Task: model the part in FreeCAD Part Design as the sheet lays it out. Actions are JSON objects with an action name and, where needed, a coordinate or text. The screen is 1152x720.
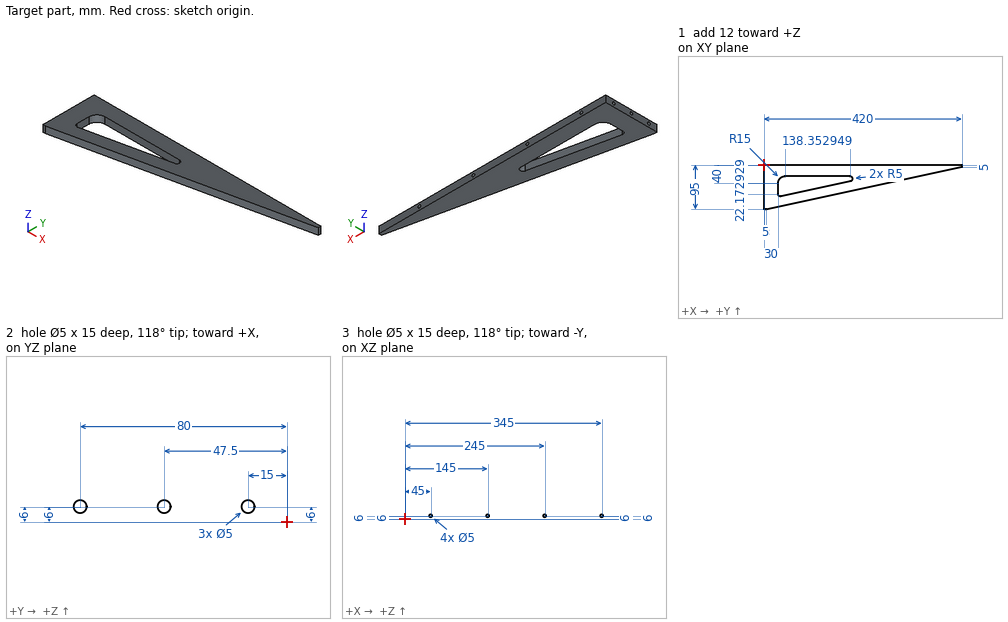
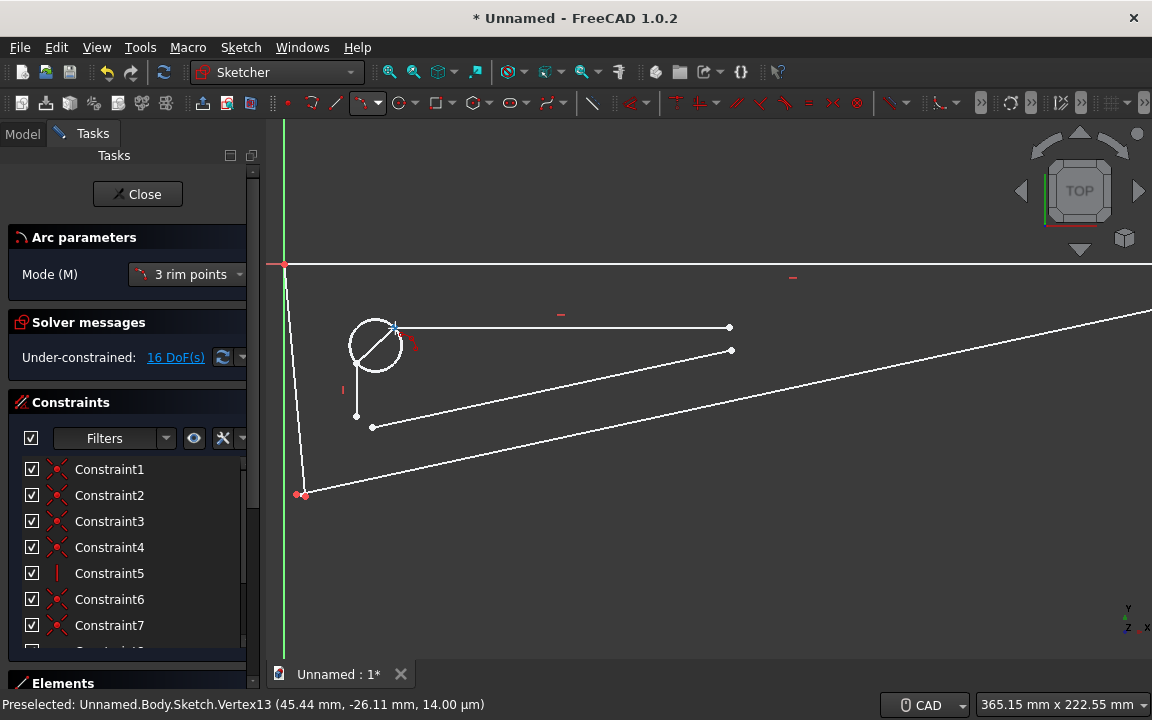
{"action": "scroll", "coordinate": [368, 336], "scroll_direction": "up", "scroll_amount": 2}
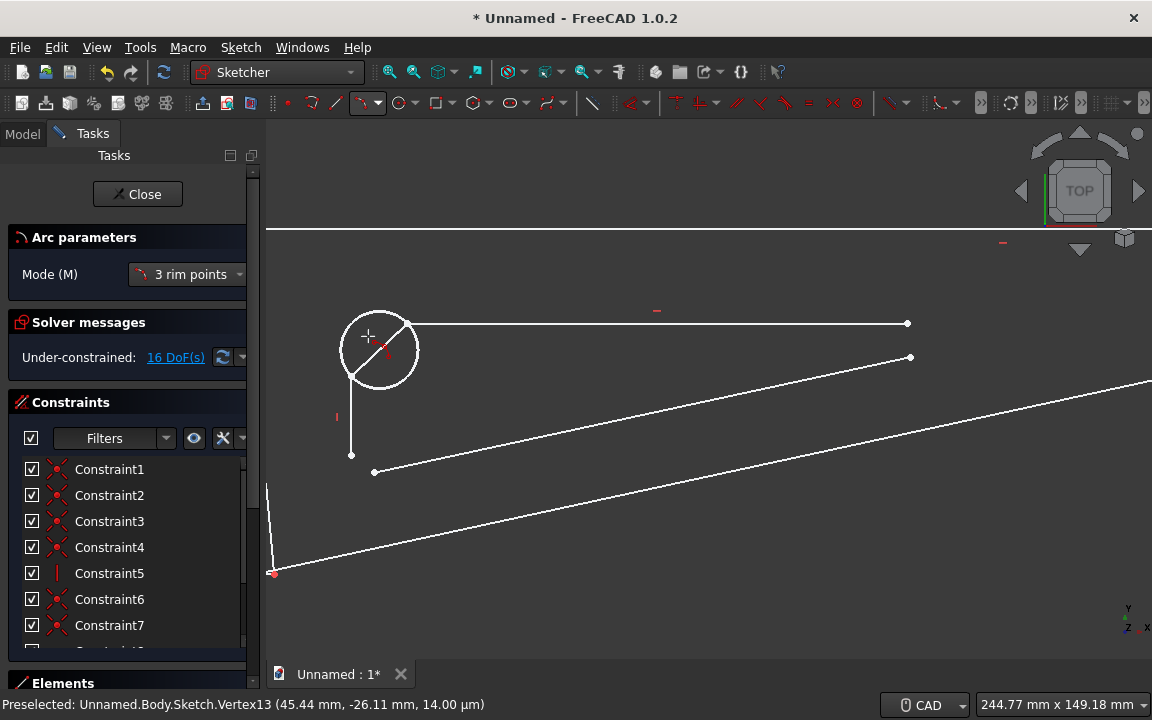
{"action": "left_click", "coordinate": [368, 335]}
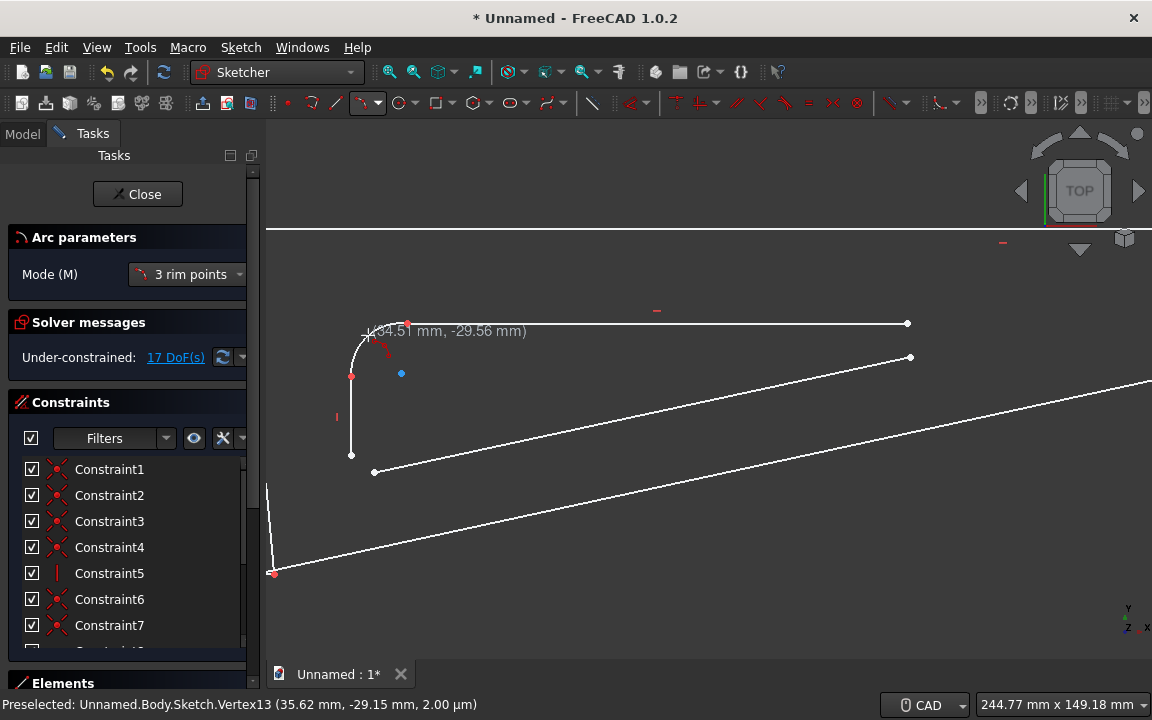
{"action": "left_click", "coordinate": [907, 324]}
{"action": "left_click", "coordinate": [911, 357]}
{"action": "left_click", "coordinate": [925, 336]}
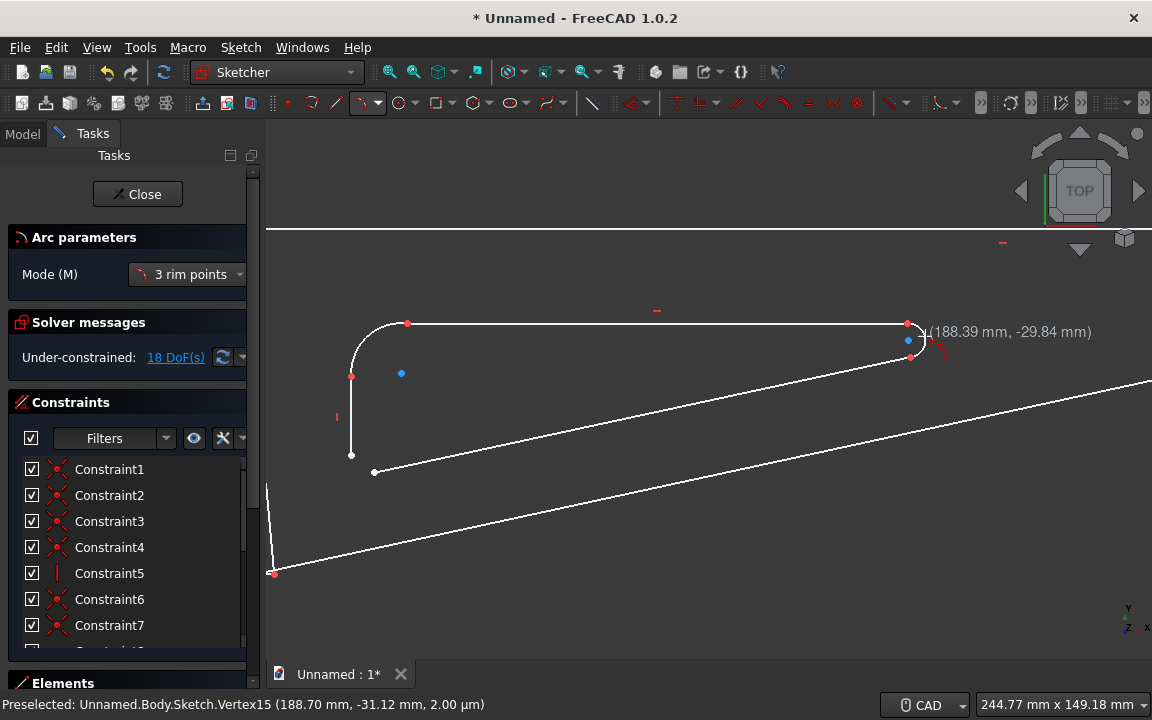
{"action": "left_click", "coordinate": [374, 473]}
{"action": "left_click", "coordinate": [351, 456]}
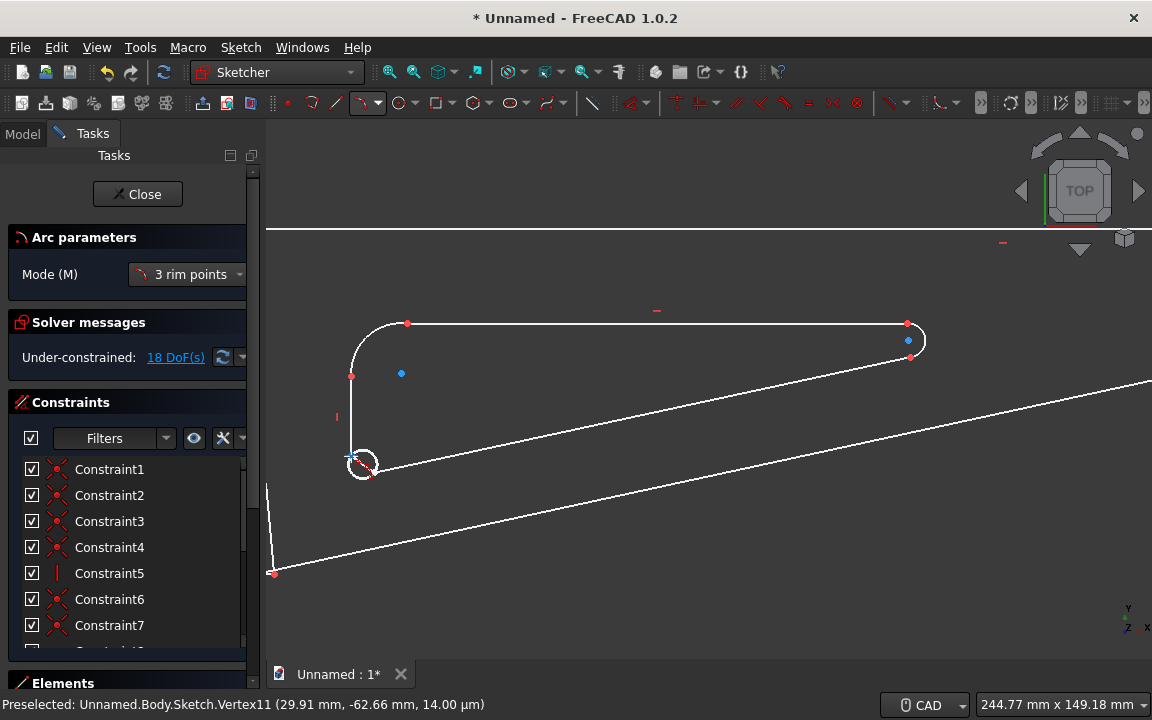
{"action": "scroll", "coordinate": [358, 468], "scroll_direction": "up", "scroll_amount": 5}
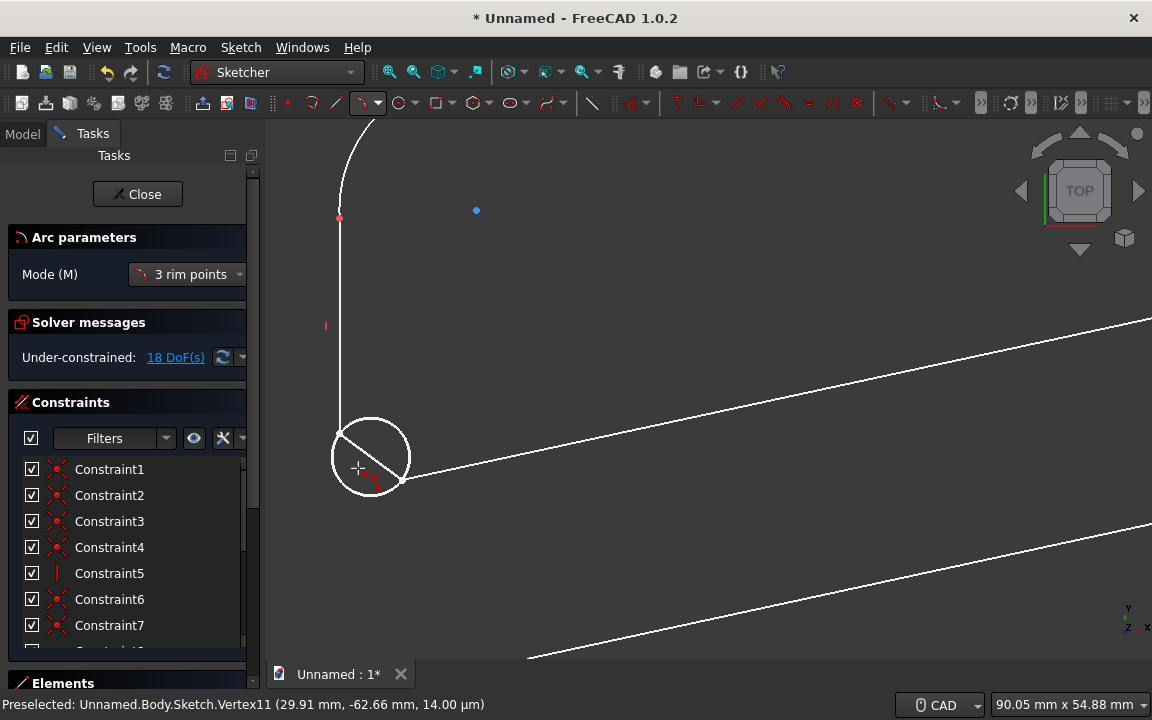
{"action": "left_click", "coordinate": [359, 467]}
{"action": "key", "text": "Escape"}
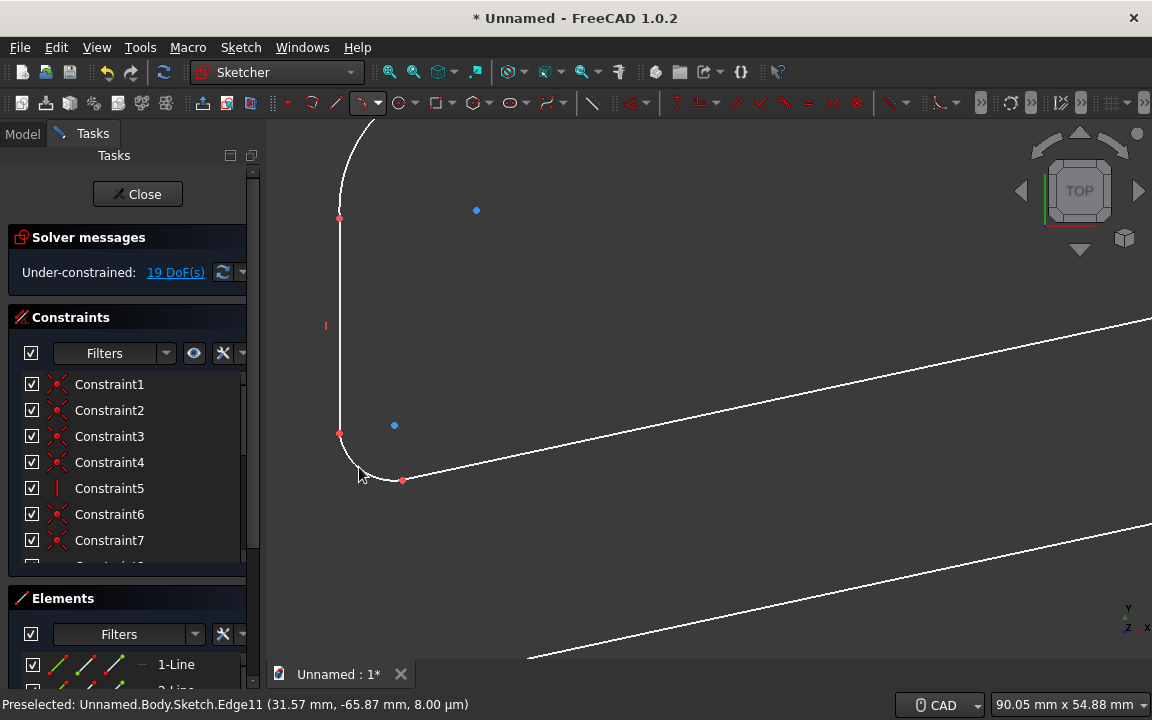
{"action": "scroll", "coordinate": [457, 402], "scroll_direction": "down", "scroll_amount": 11}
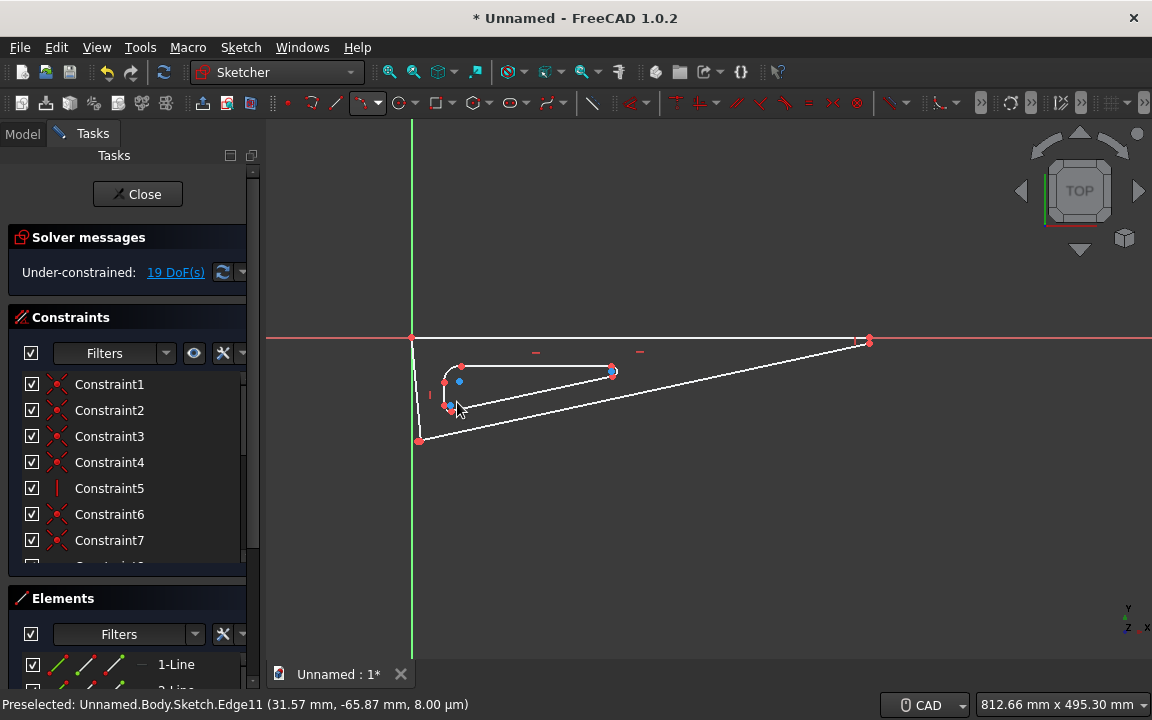
{"action": "scroll", "coordinate": [444, 399], "scroll_direction": "up", "scroll_amount": 4}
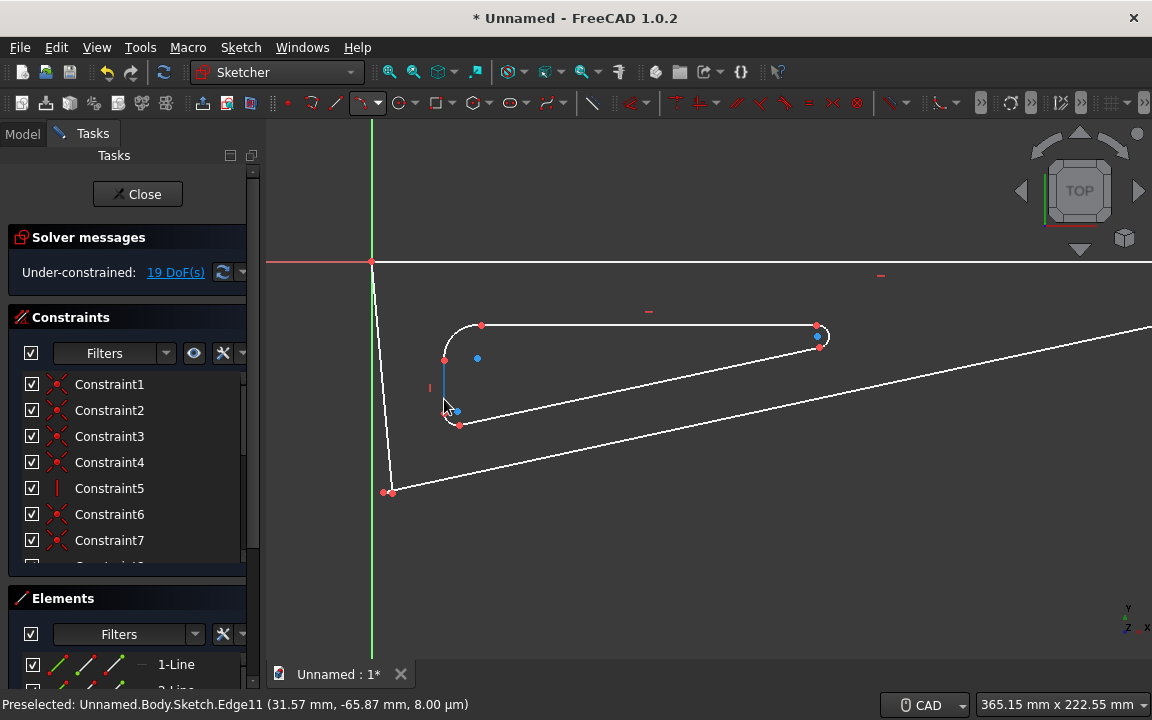
{"action": "left_click", "coordinate": [444, 398]}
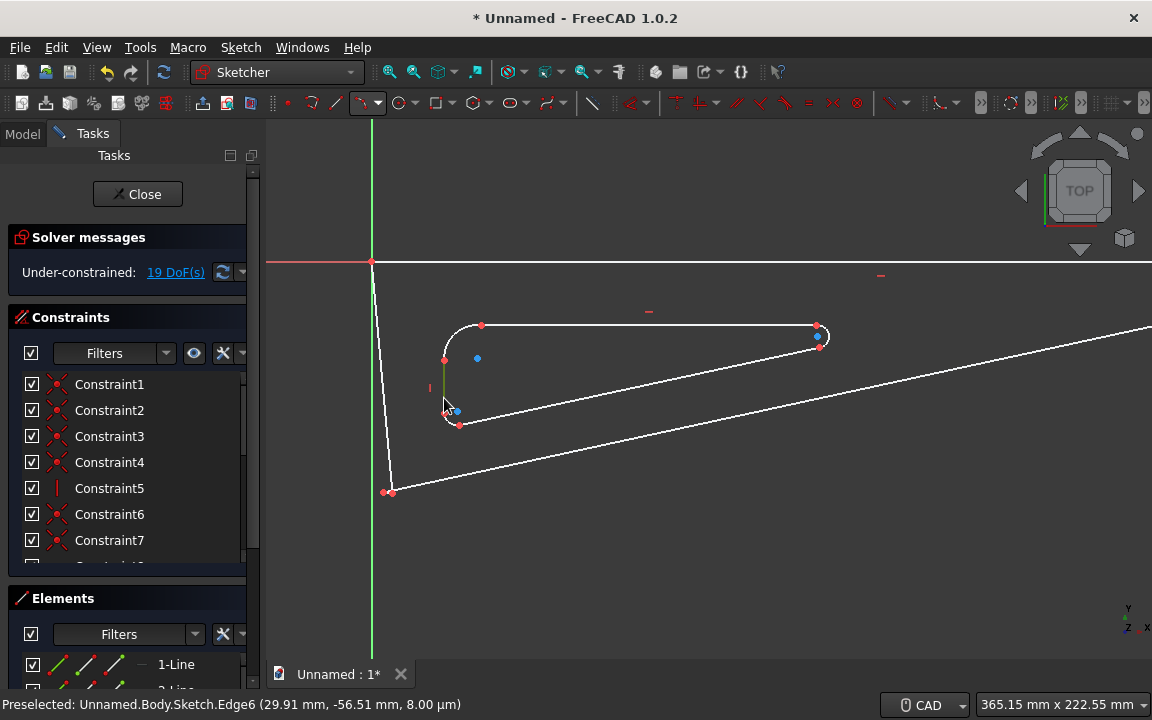
{"action": "left_click", "coordinate": [465, 328]}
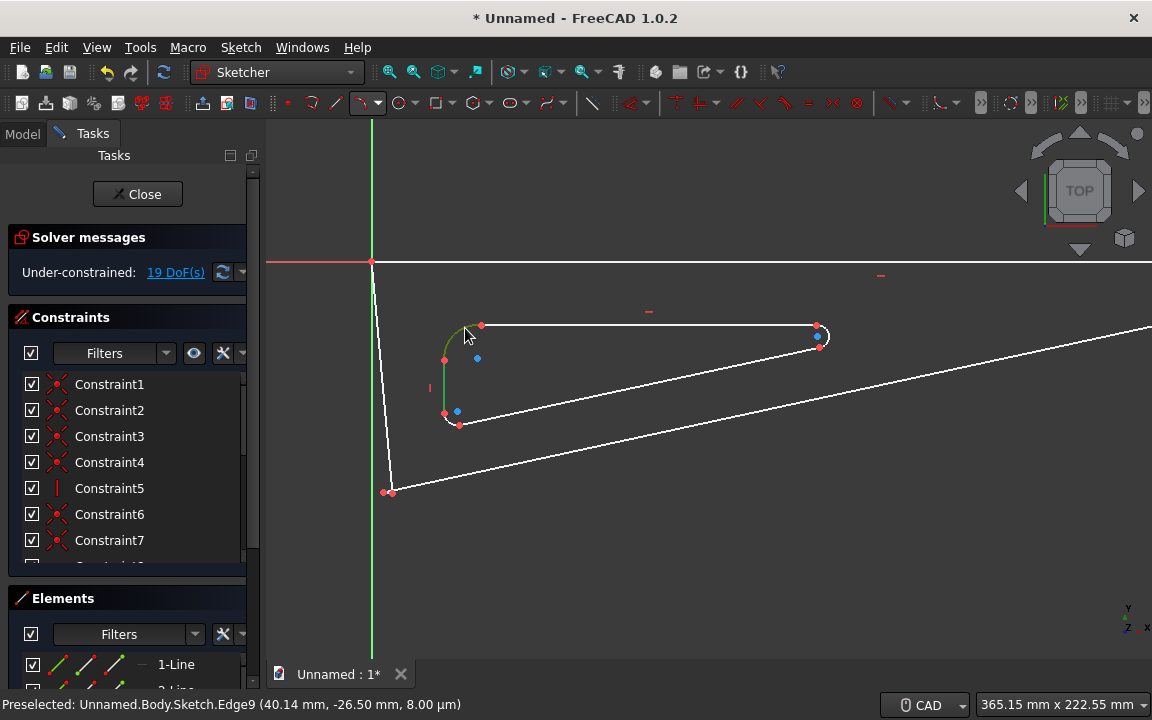
{"action": "left_click", "coordinate": [786, 104]}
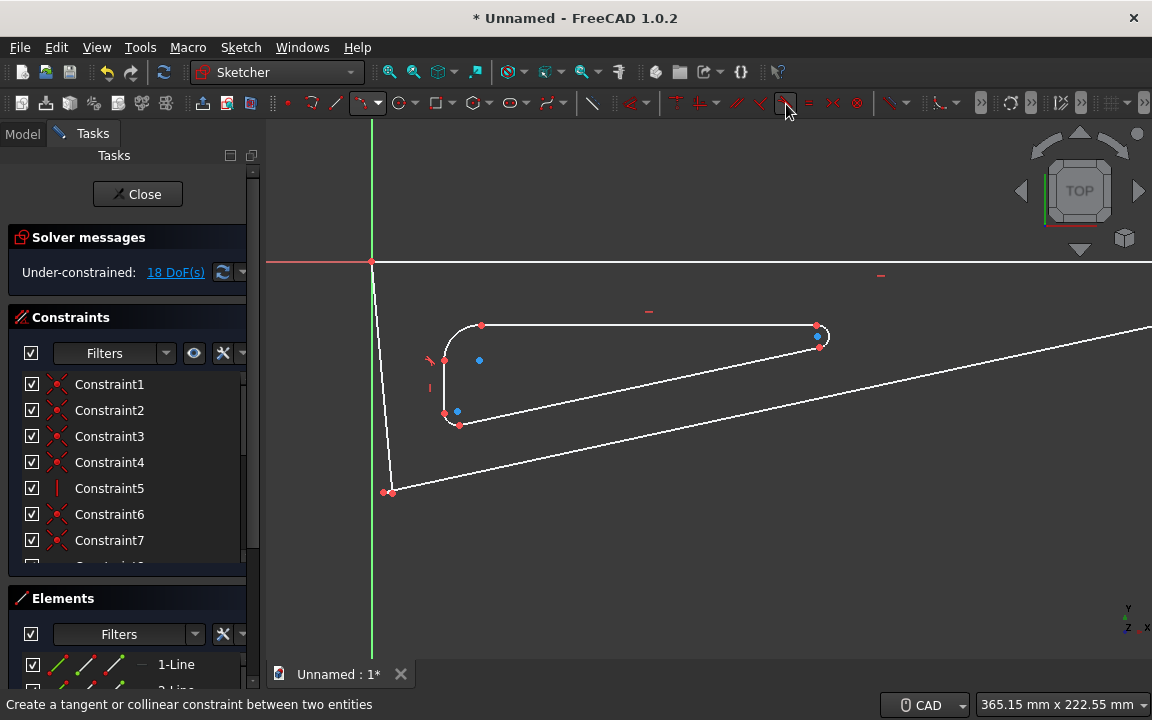
{"action": "left_click", "coordinate": [444, 398]}